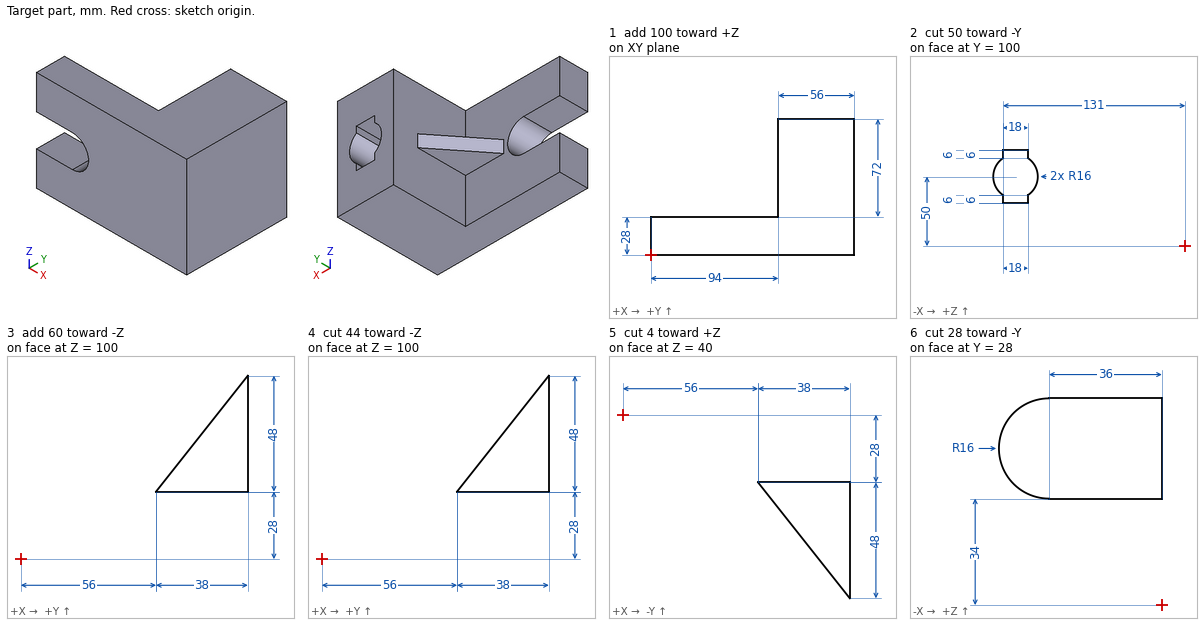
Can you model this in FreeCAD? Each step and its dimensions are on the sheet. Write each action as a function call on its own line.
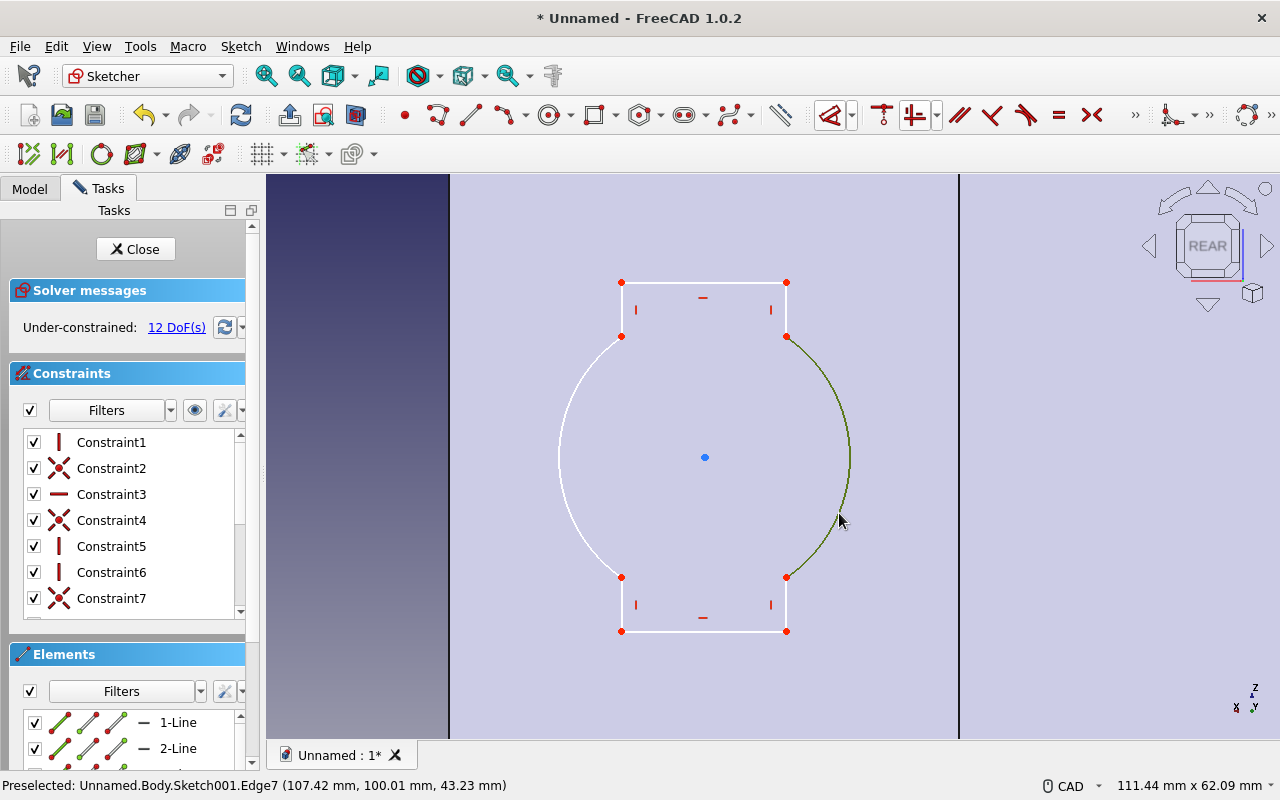
click(570, 402)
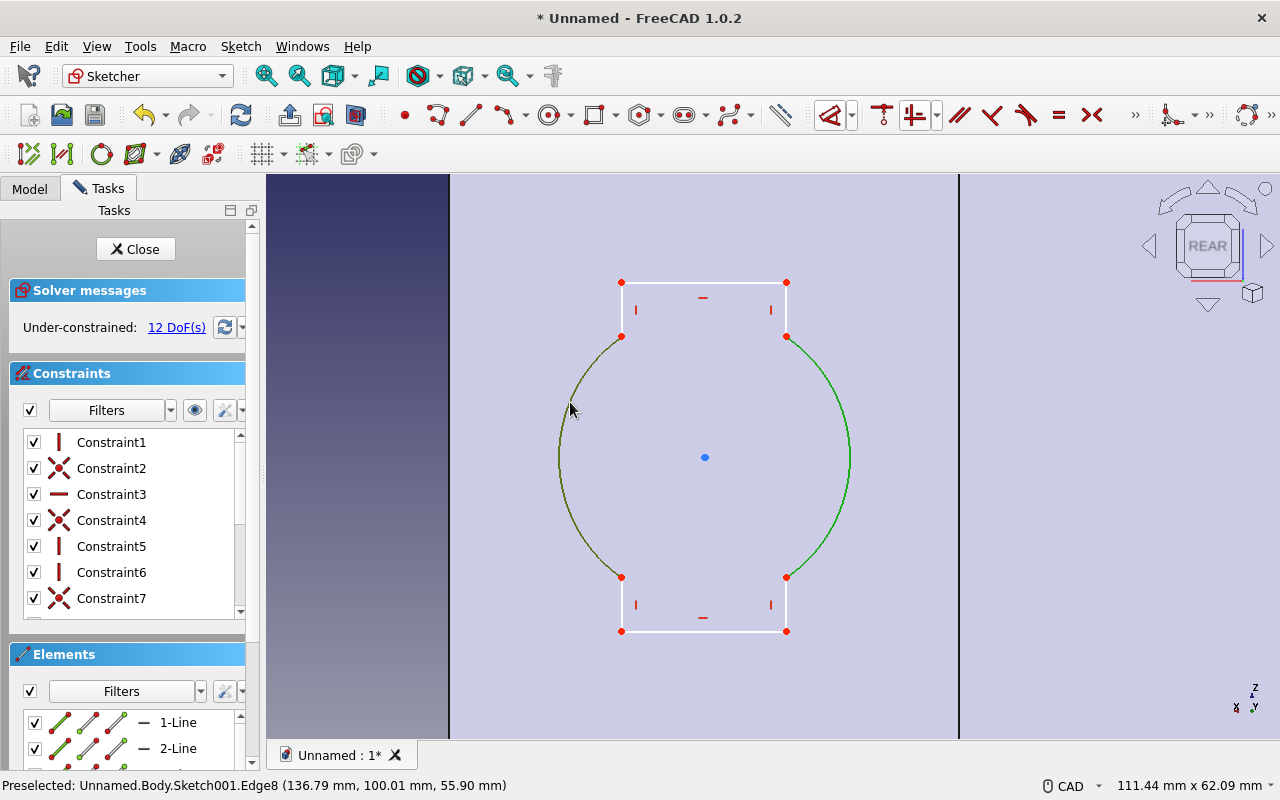
click(882, 116)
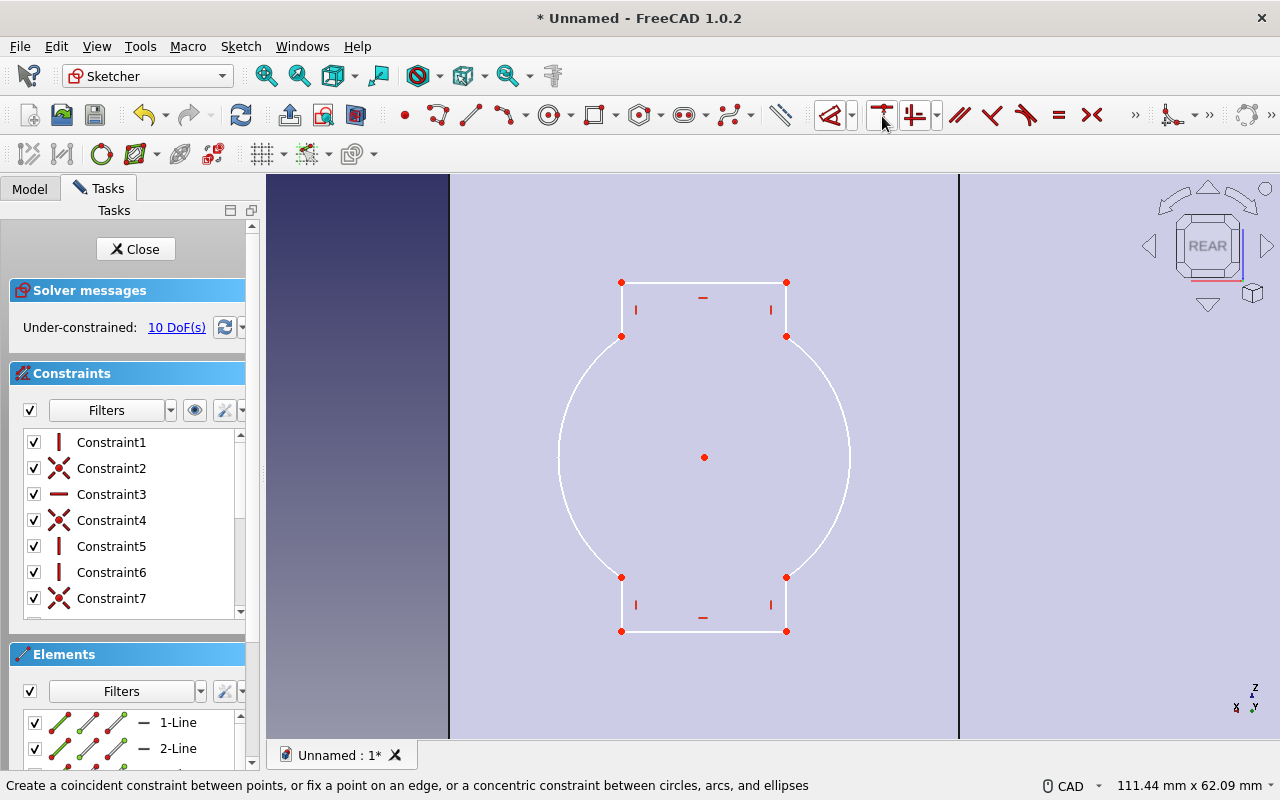
click(839, 513)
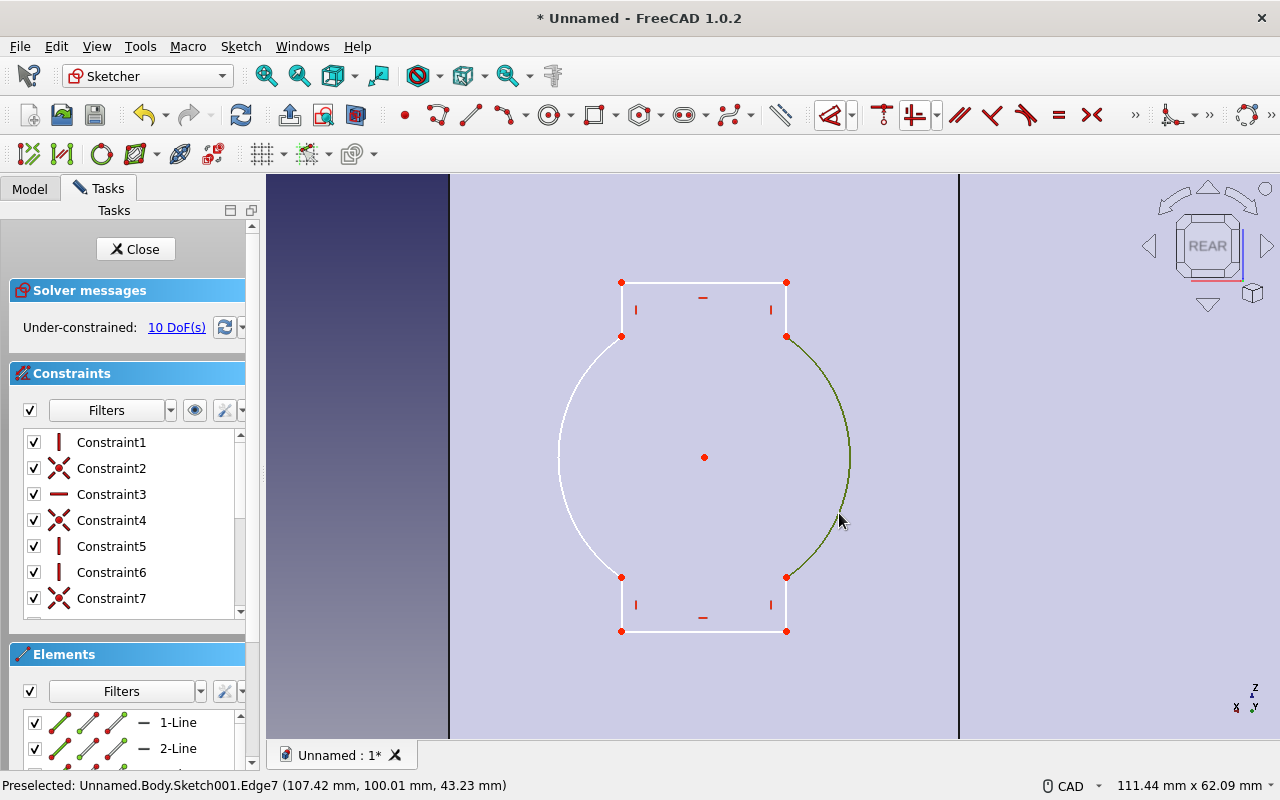
click(569, 402)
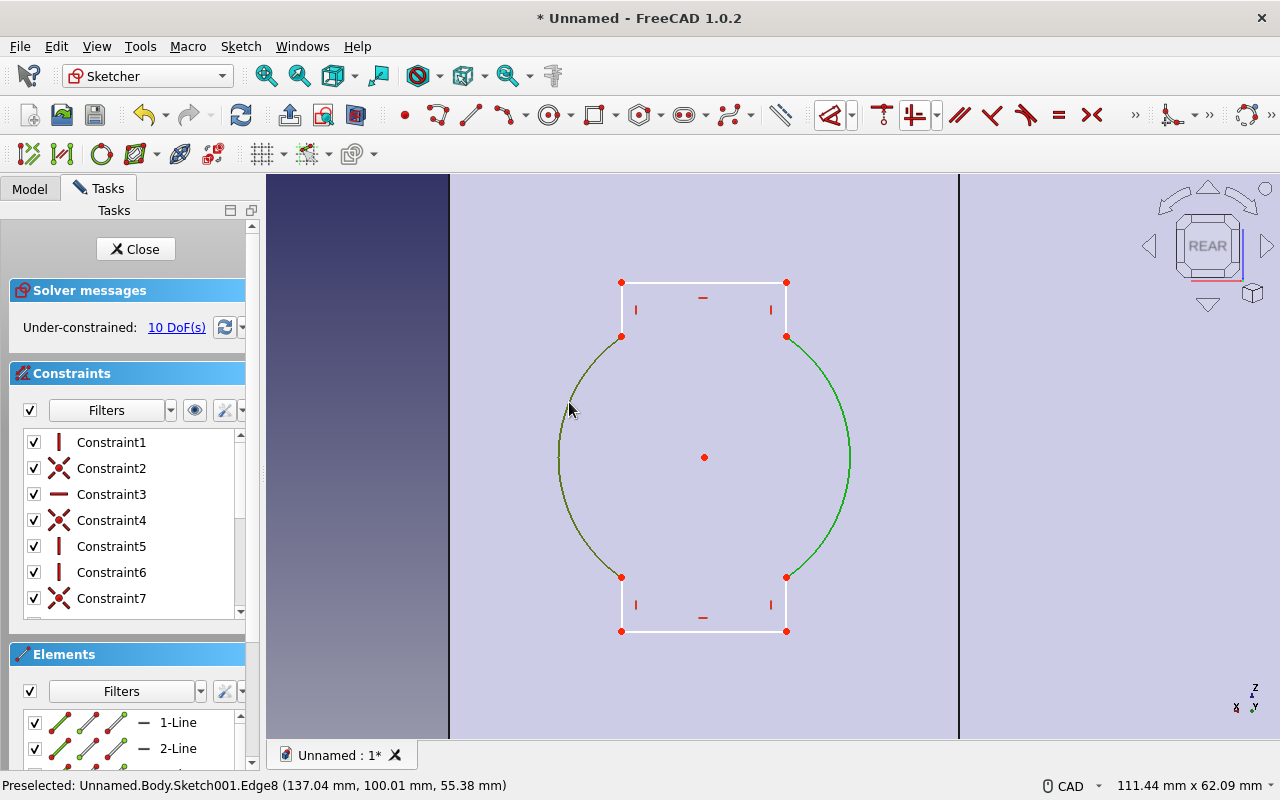
click(1059, 116)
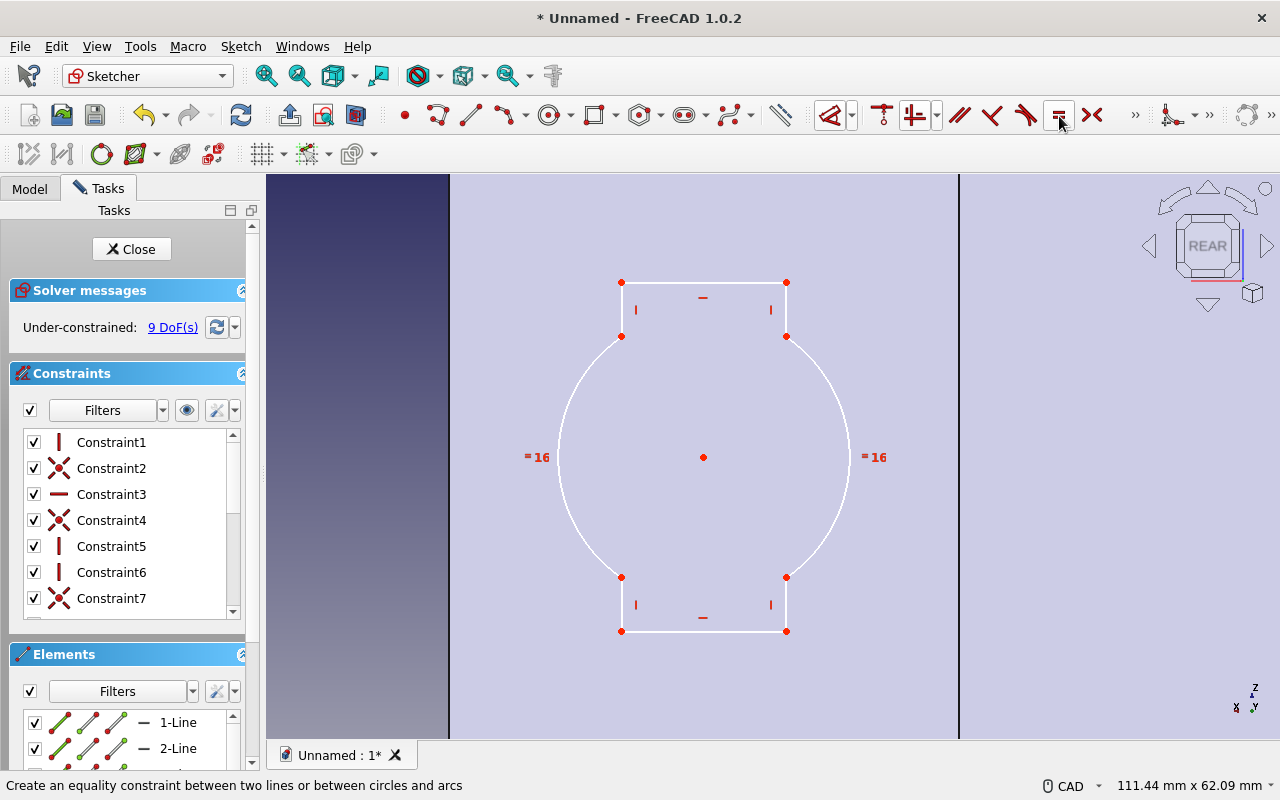
click(839, 513)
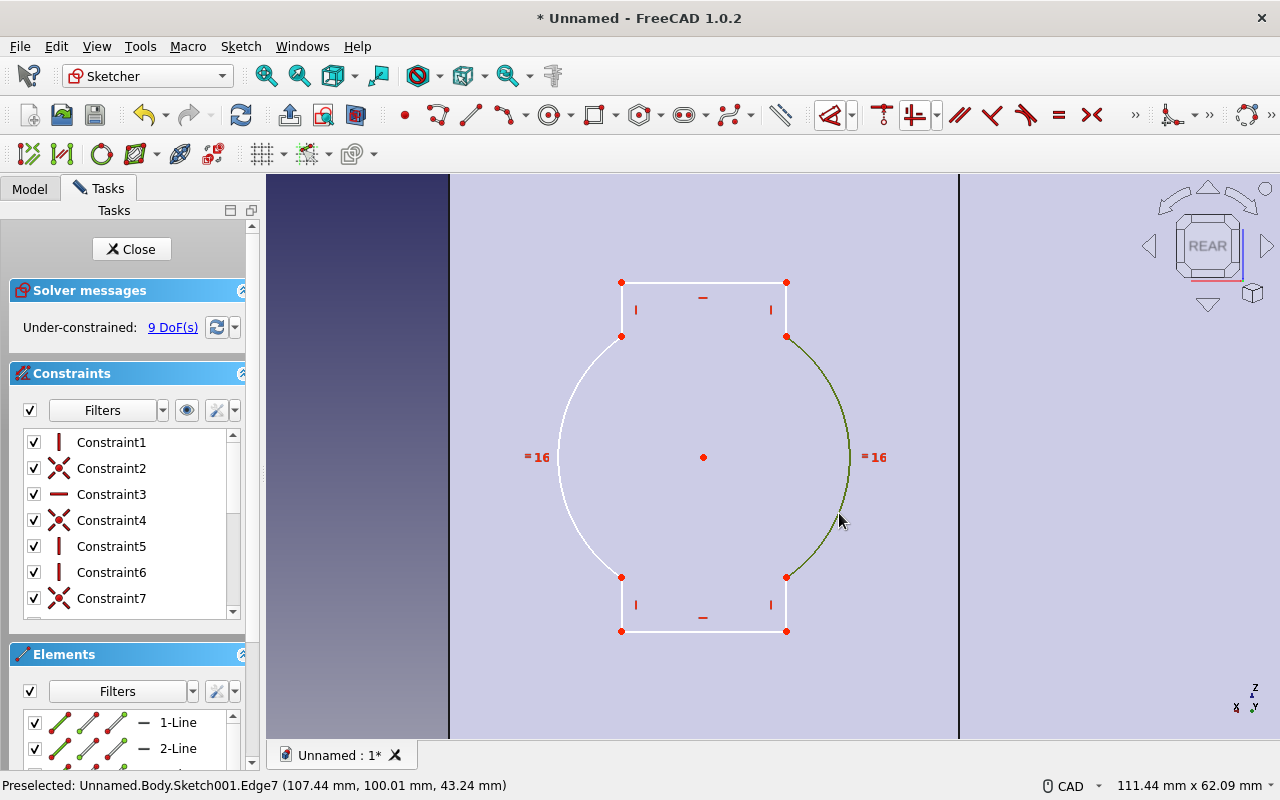
key(k)
key(r)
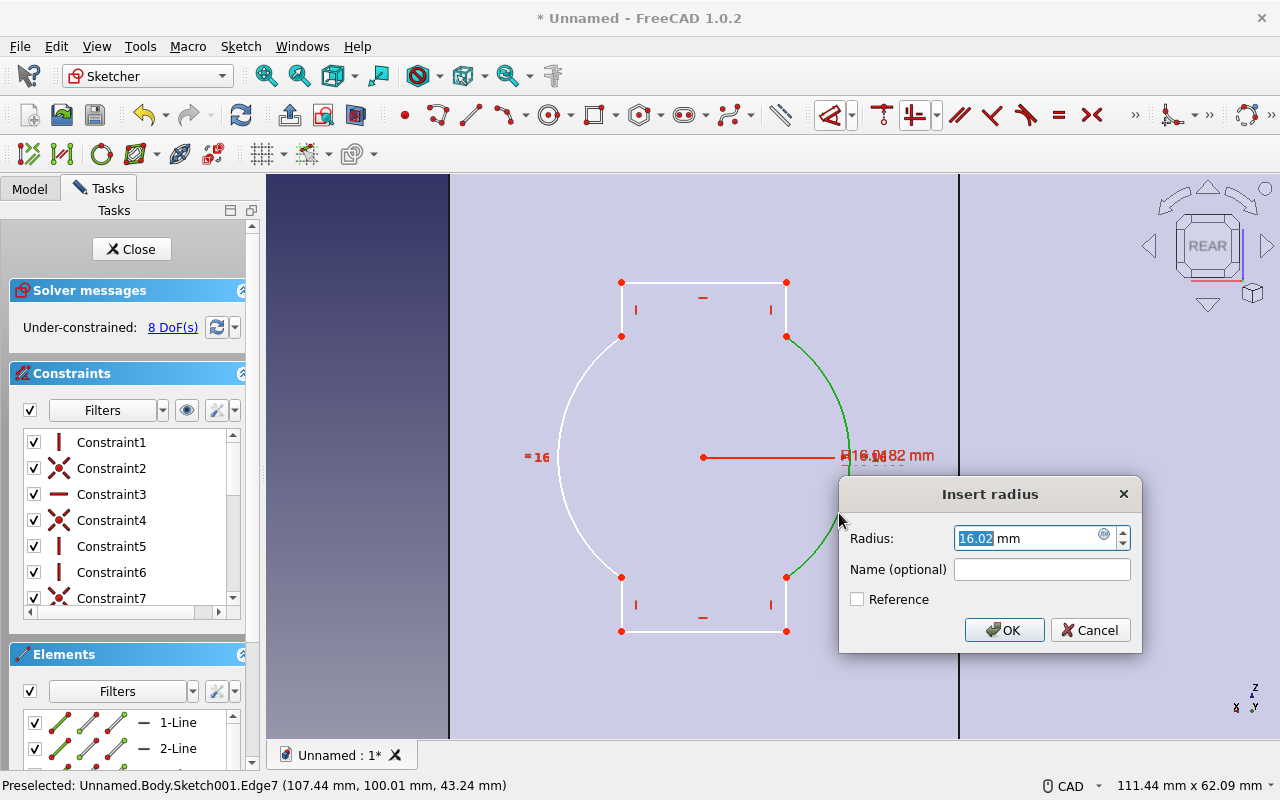
text(16)
key(Return)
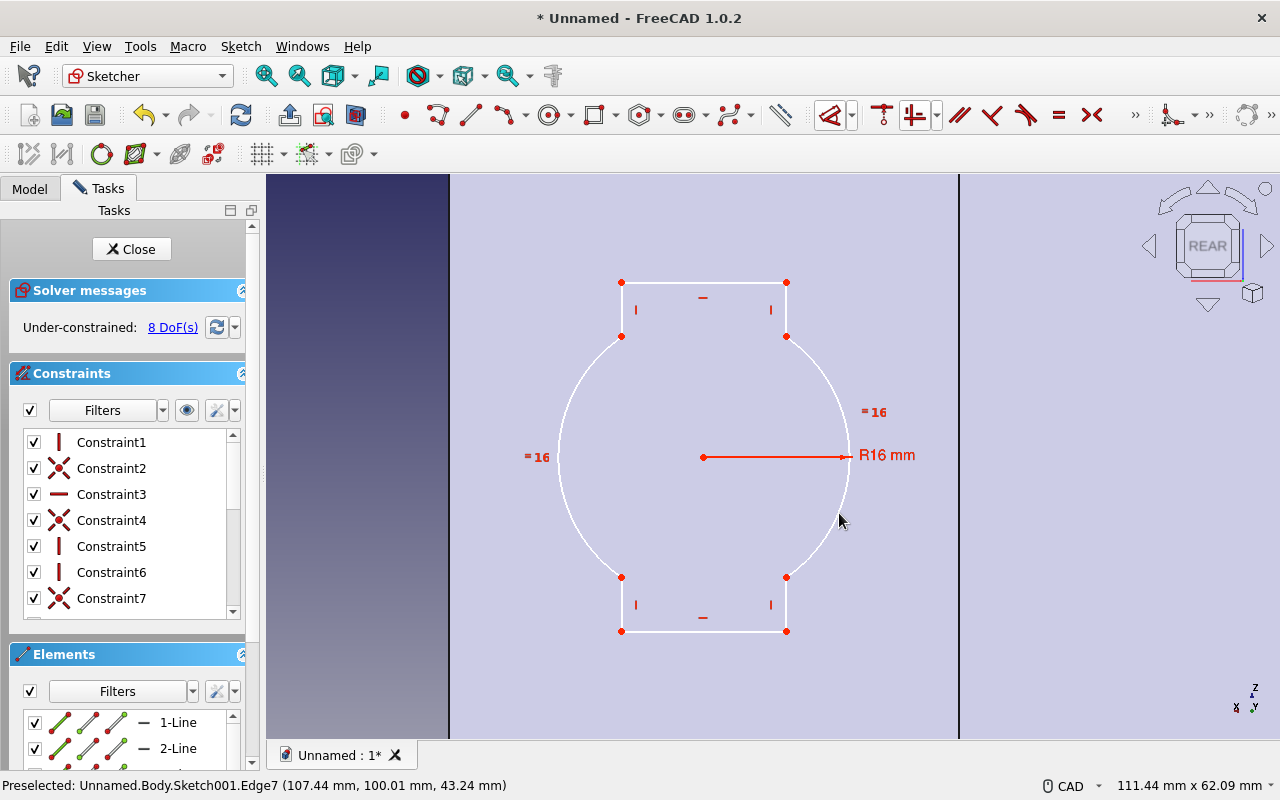
click(622, 594)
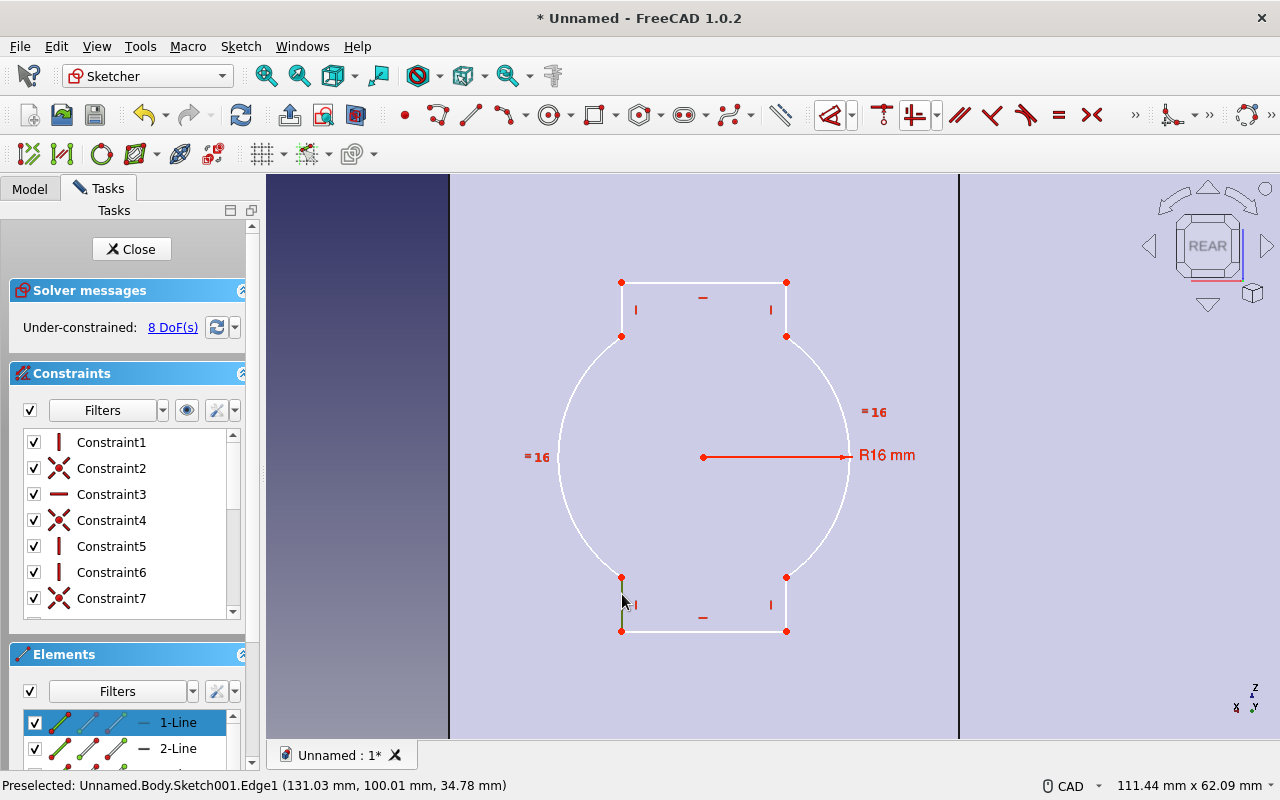
key(i)